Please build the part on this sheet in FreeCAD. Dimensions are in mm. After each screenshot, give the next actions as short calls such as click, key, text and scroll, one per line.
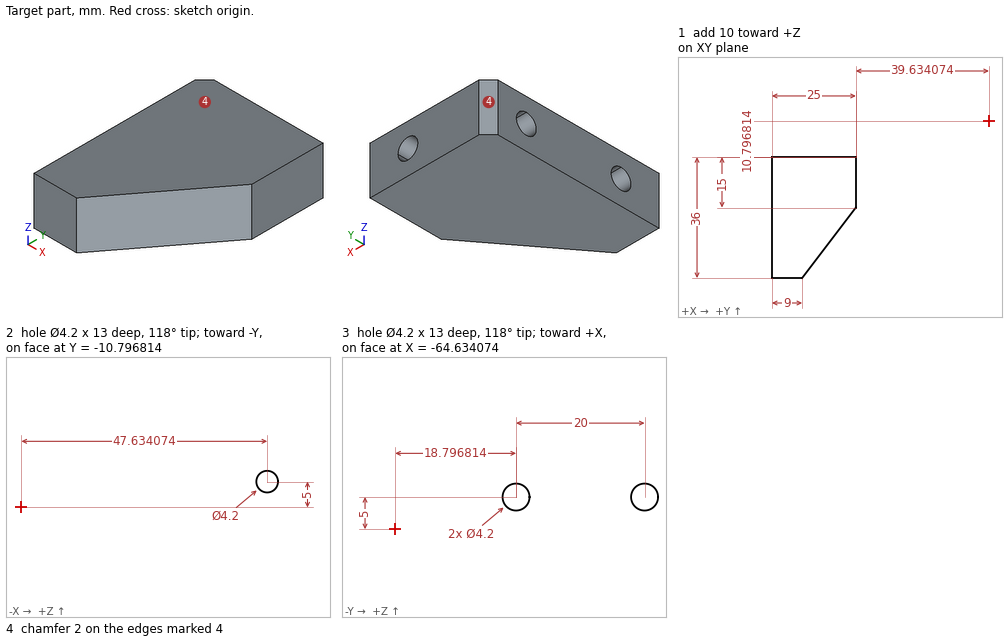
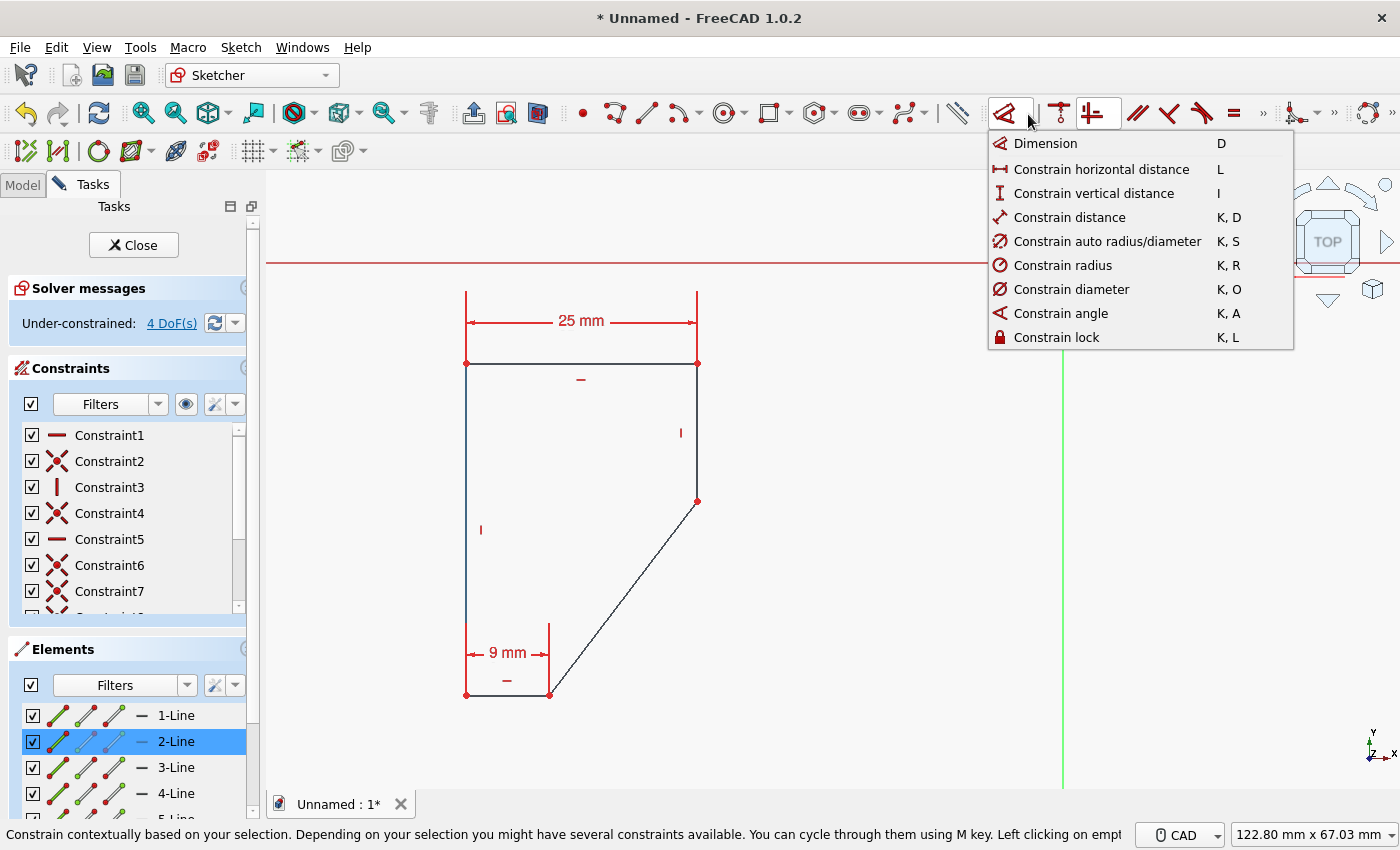
click(1141, 193)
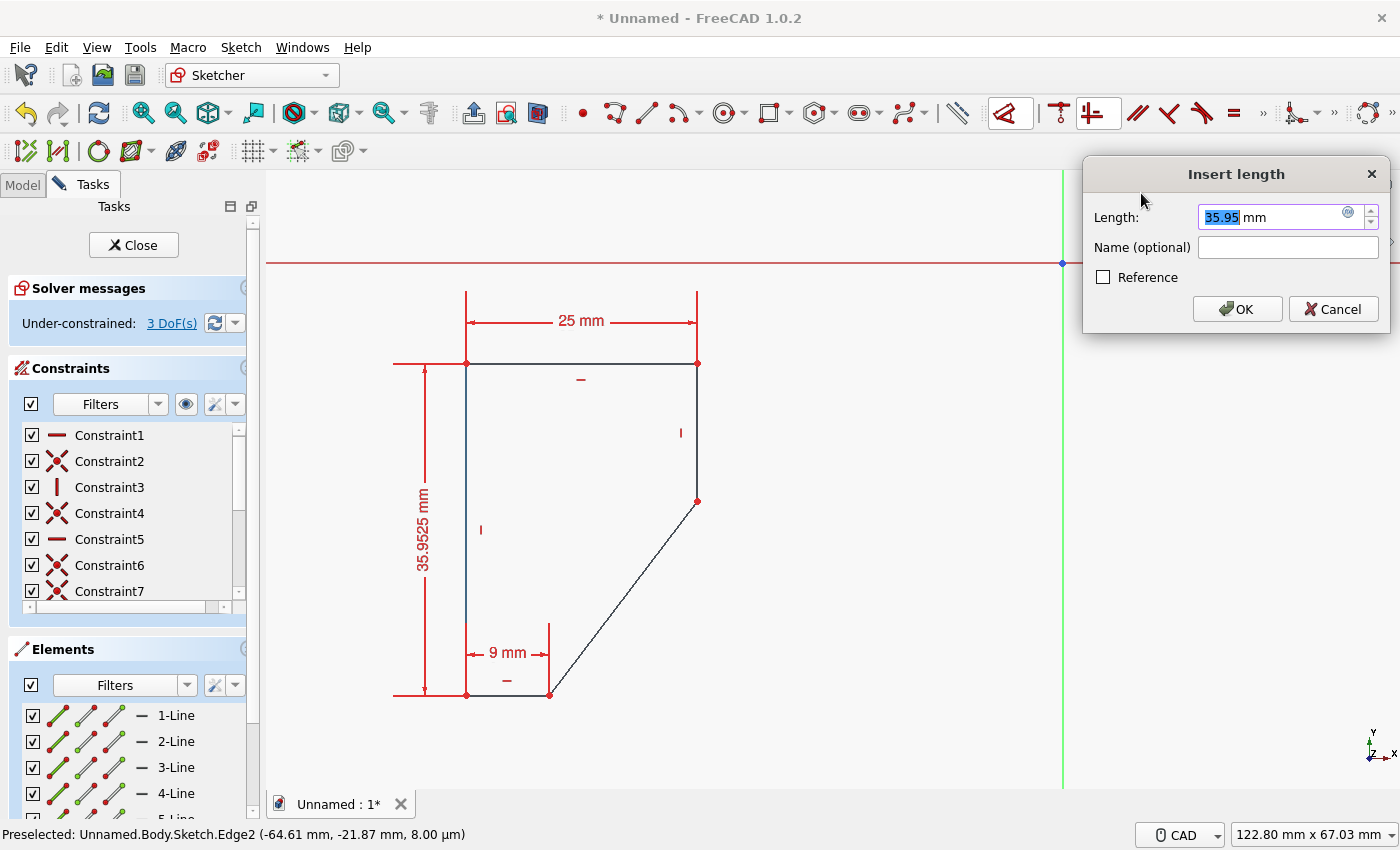
text(36)
key(Return)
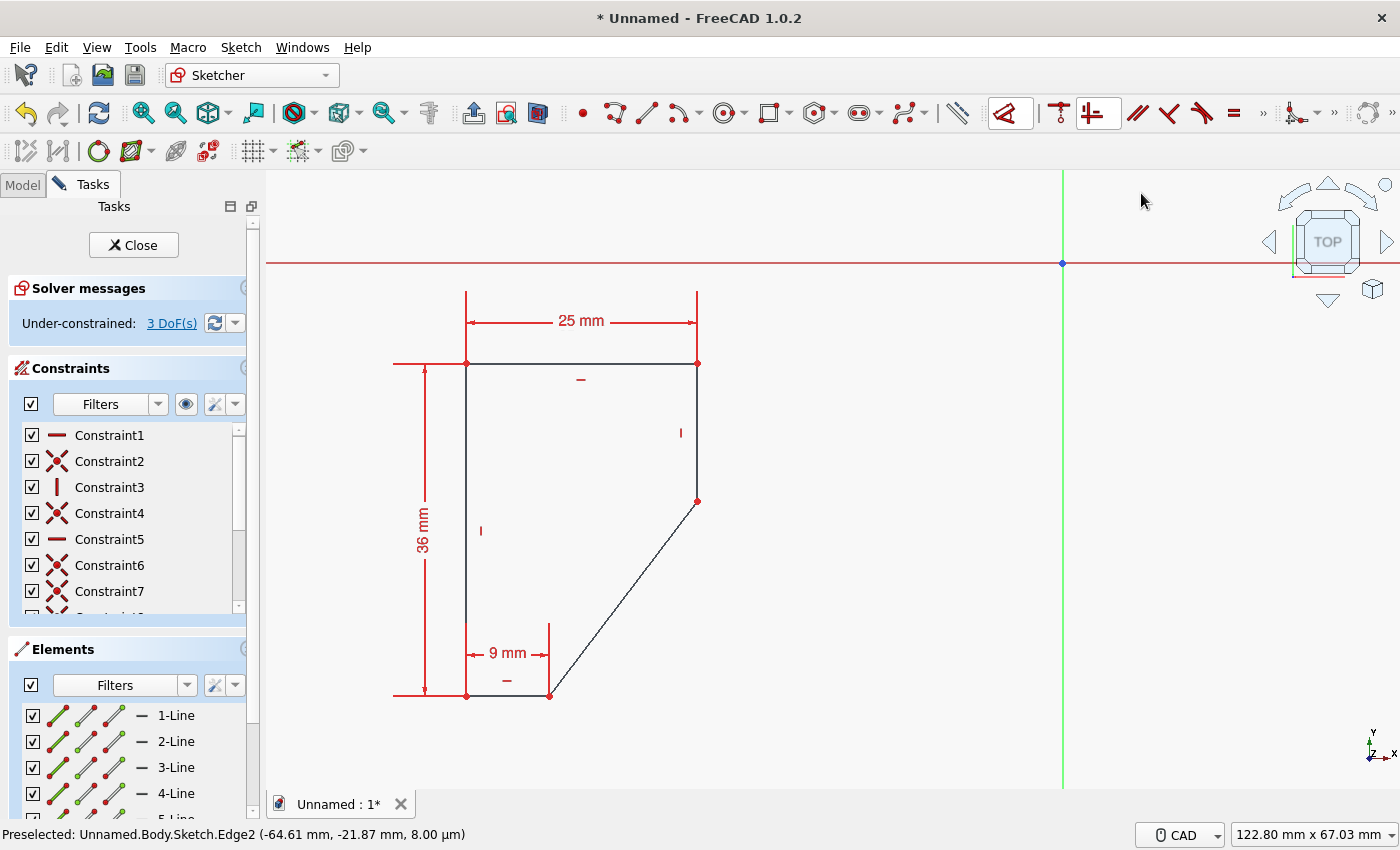
click(697, 461)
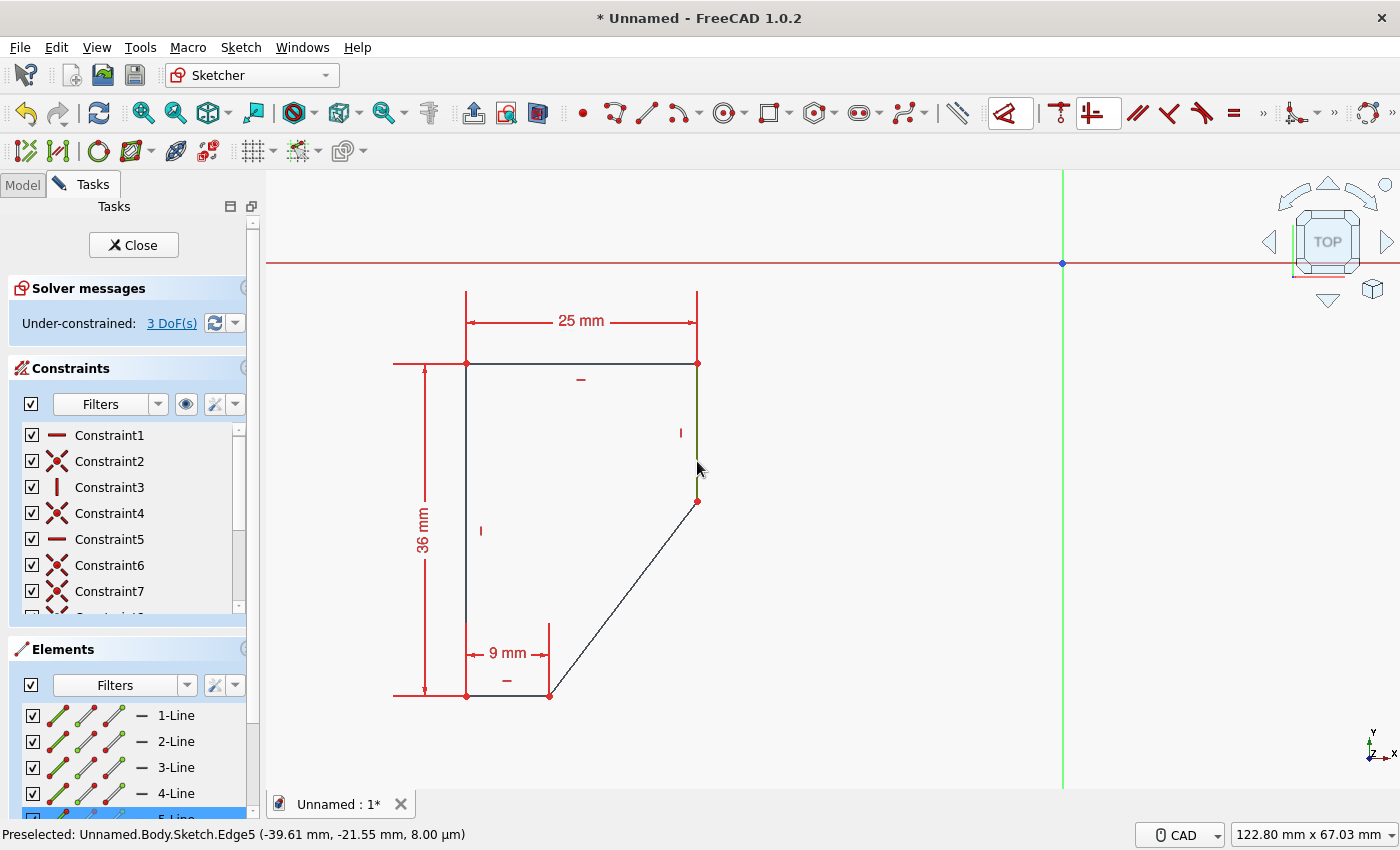
click(1028, 114)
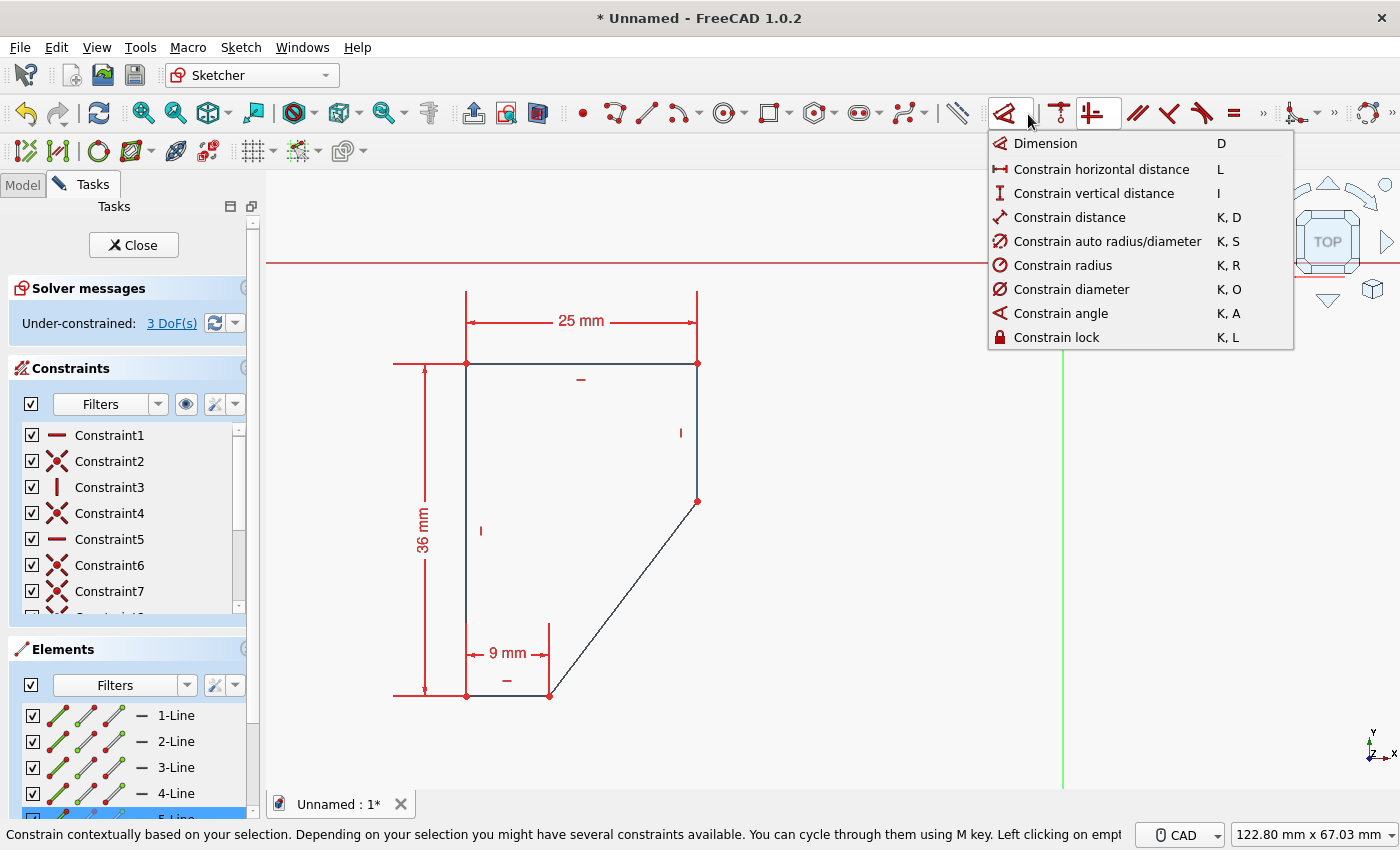
click(1141, 193)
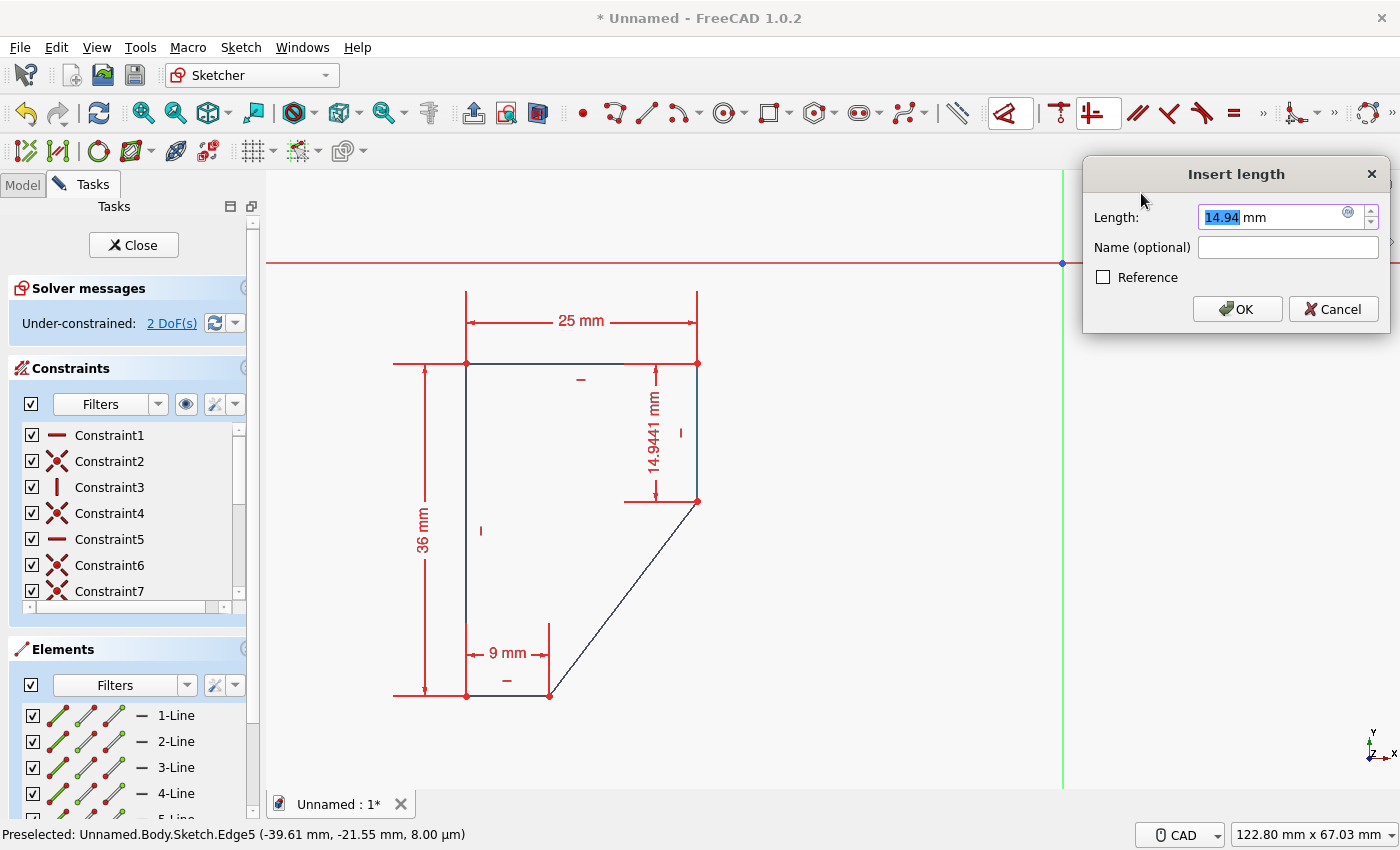
text(15)
key(Return)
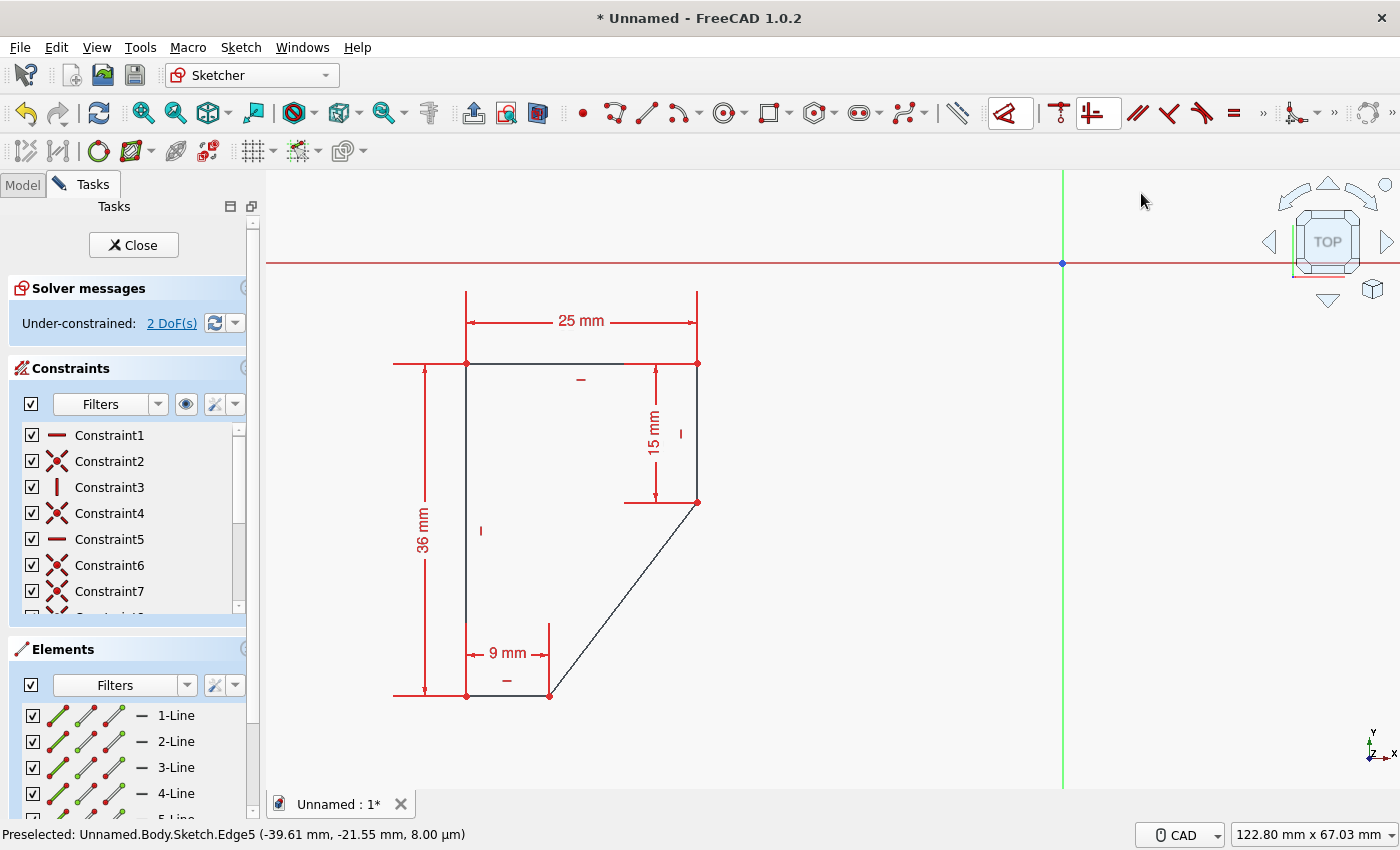
click(697, 364)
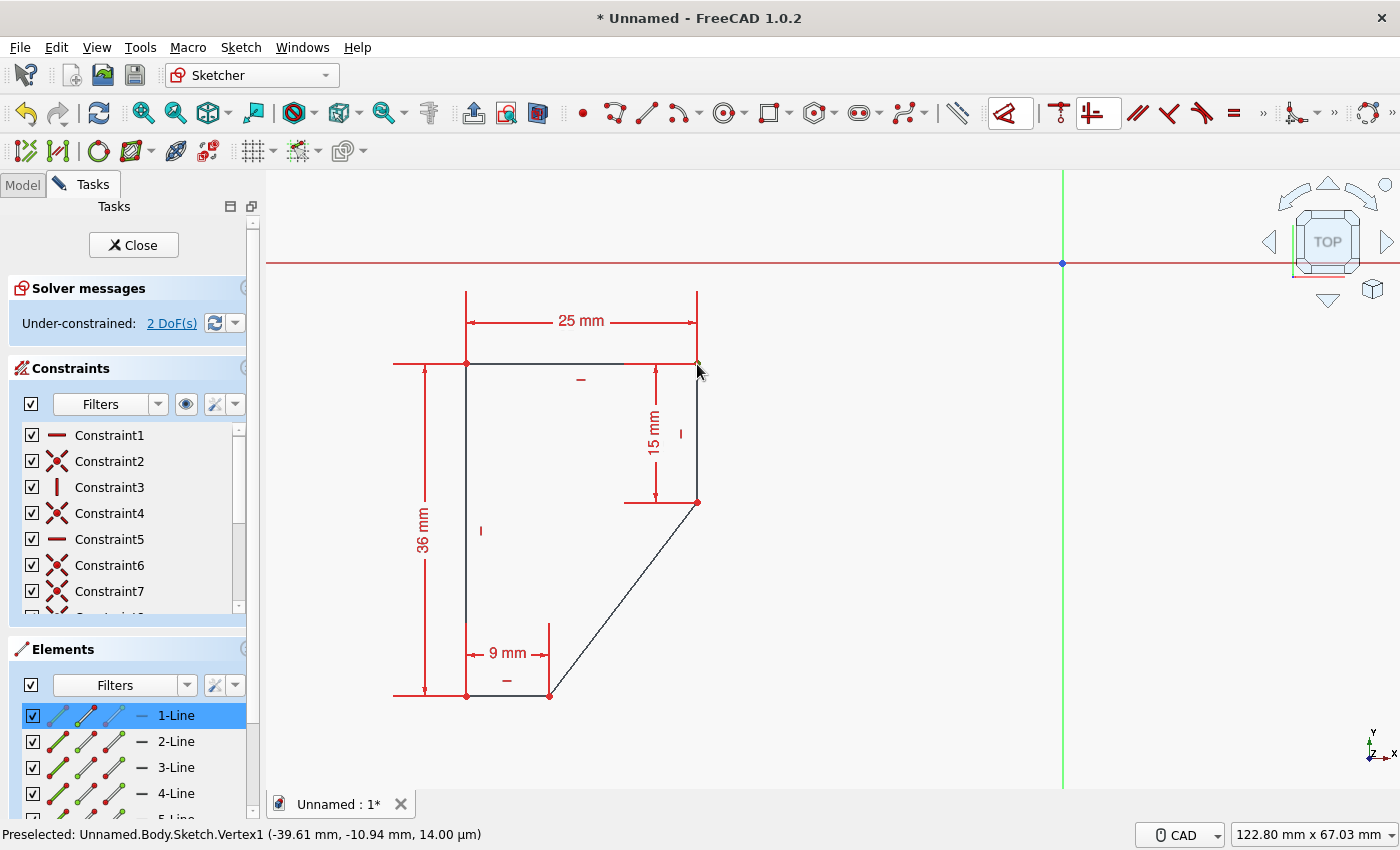
key(l)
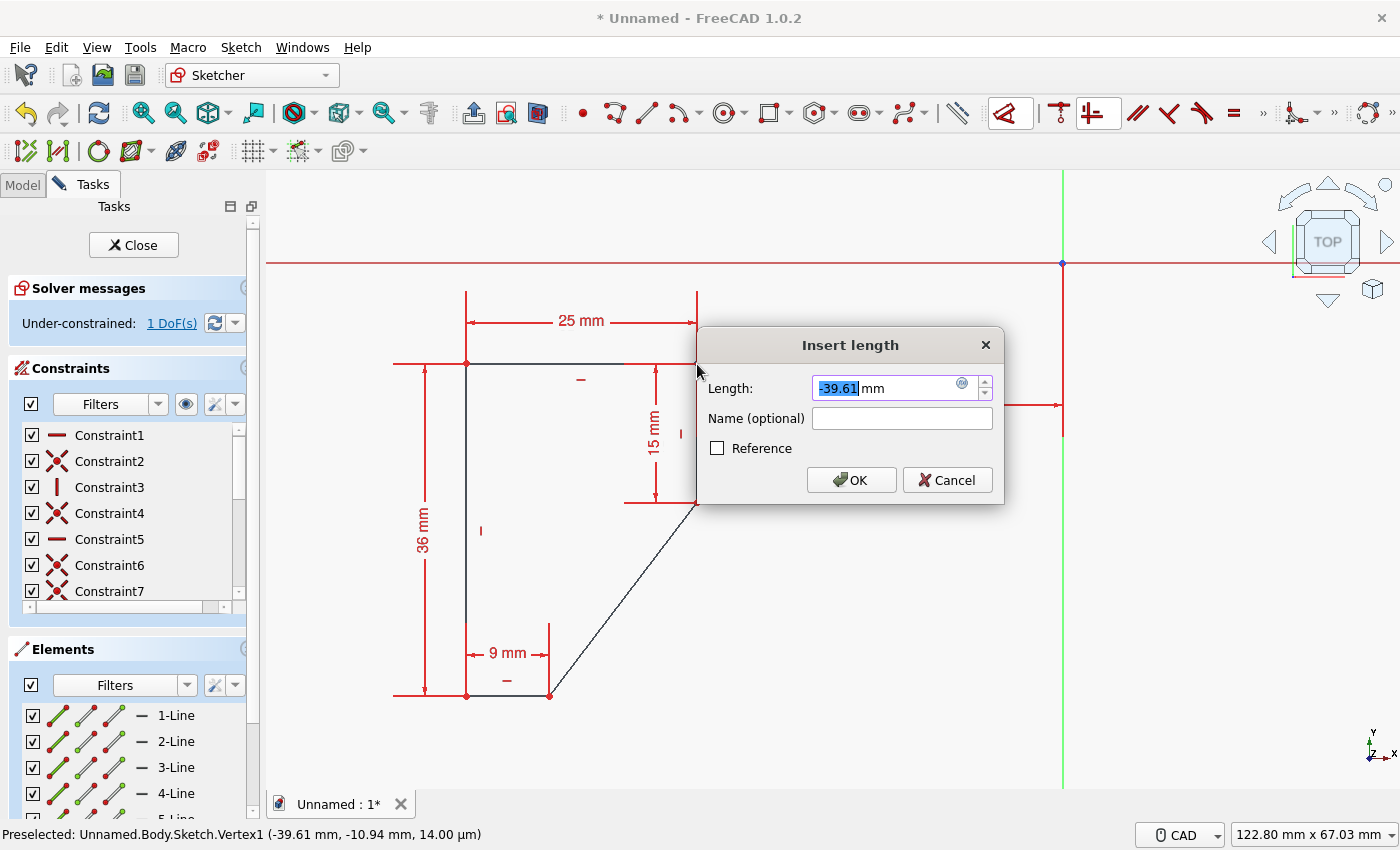
text(-39.634074)
key(Return)